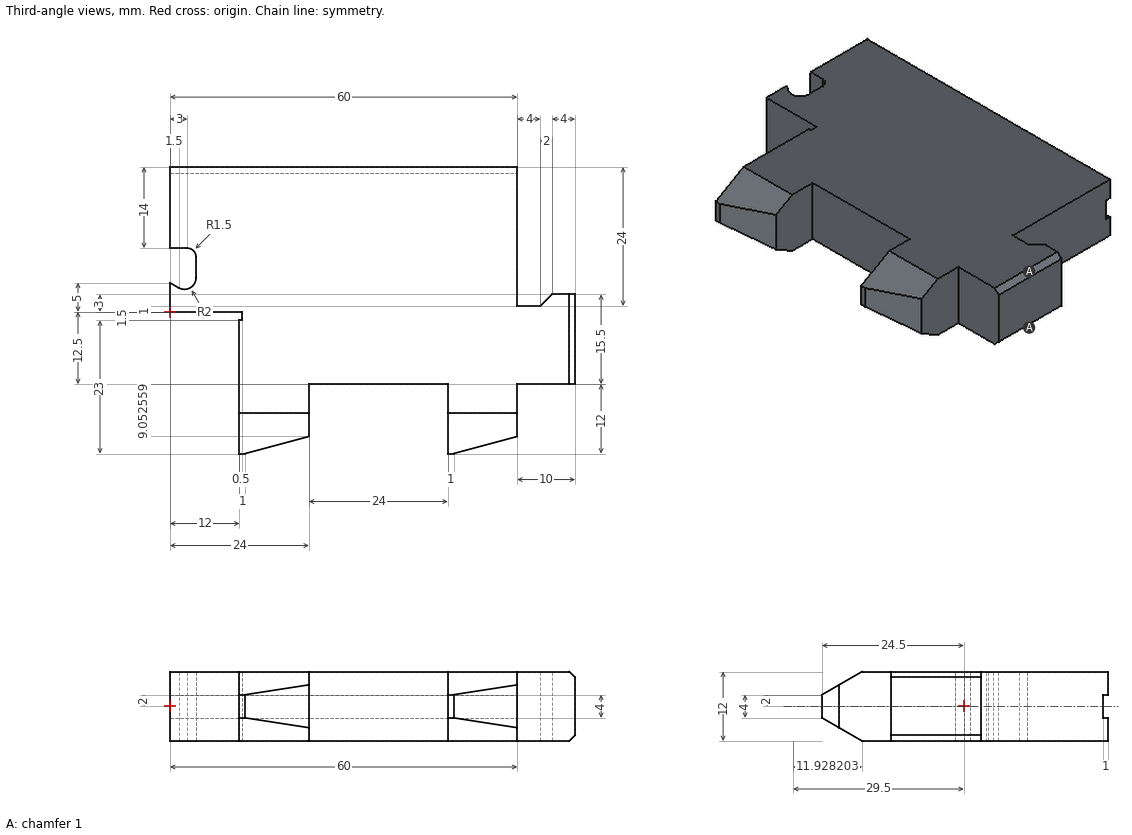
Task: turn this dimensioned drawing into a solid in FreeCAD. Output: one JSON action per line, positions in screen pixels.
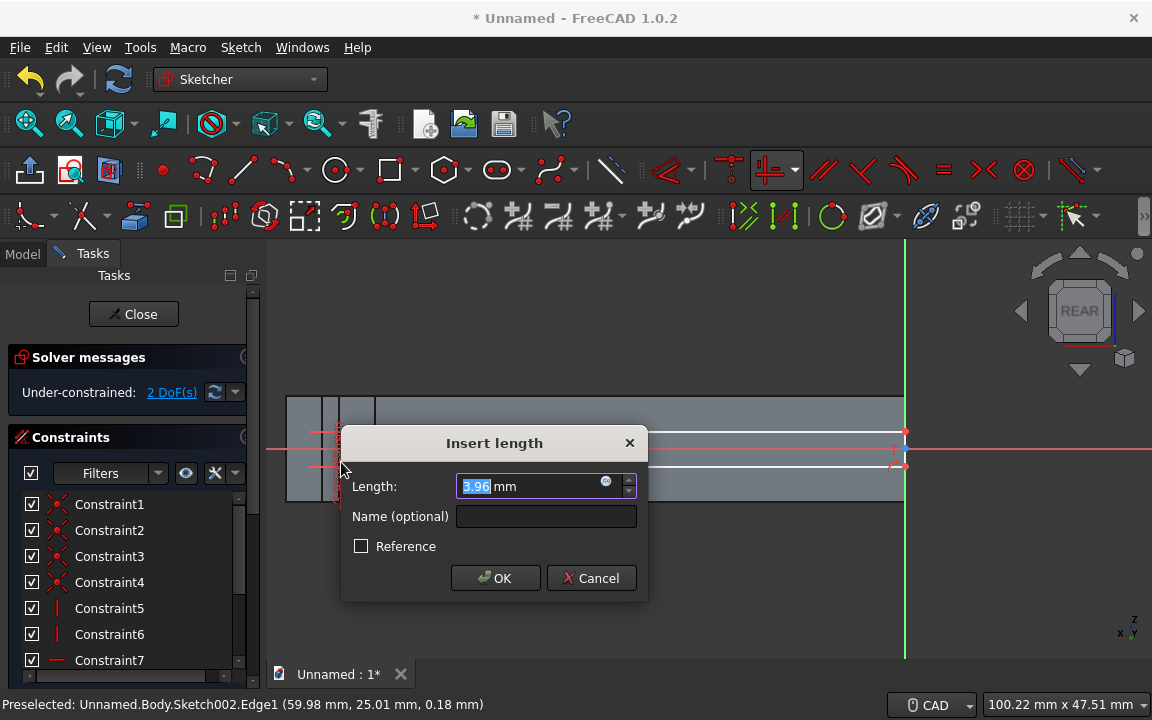
{"action": "type", "text": "4"}
{"action": "key", "text": "Return"}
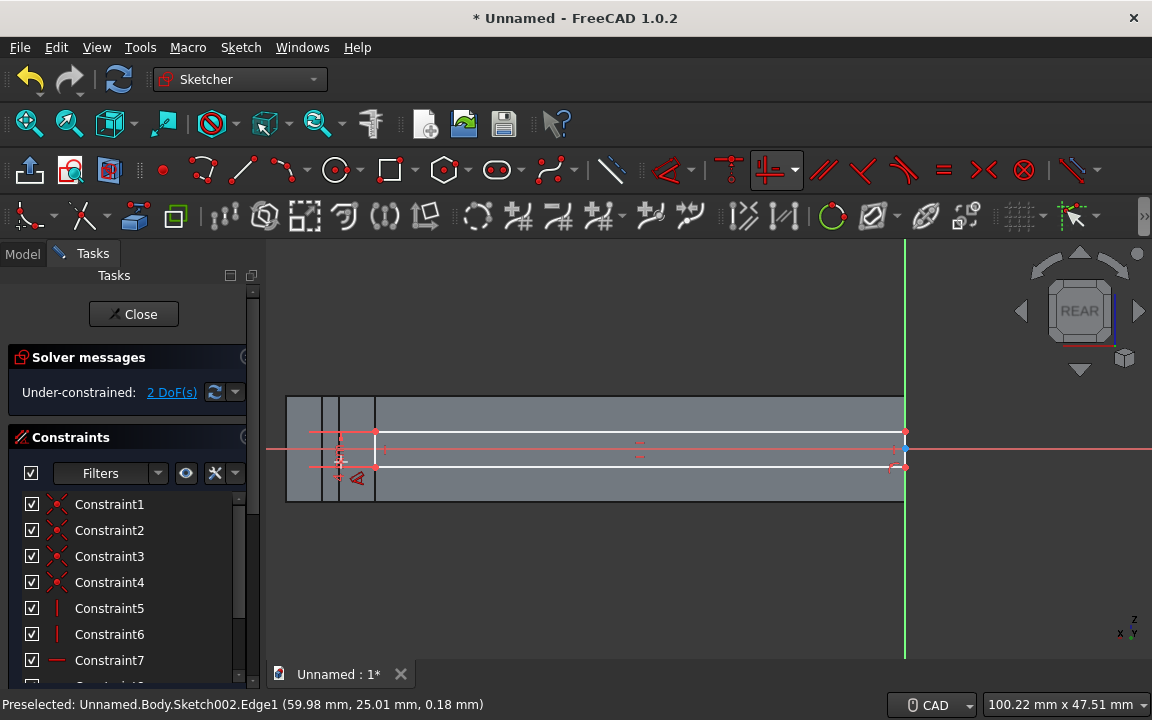
{"action": "left_click", "coordinate": [534, 467]}
{"action": "left_click", "coordinate": [640, 501]}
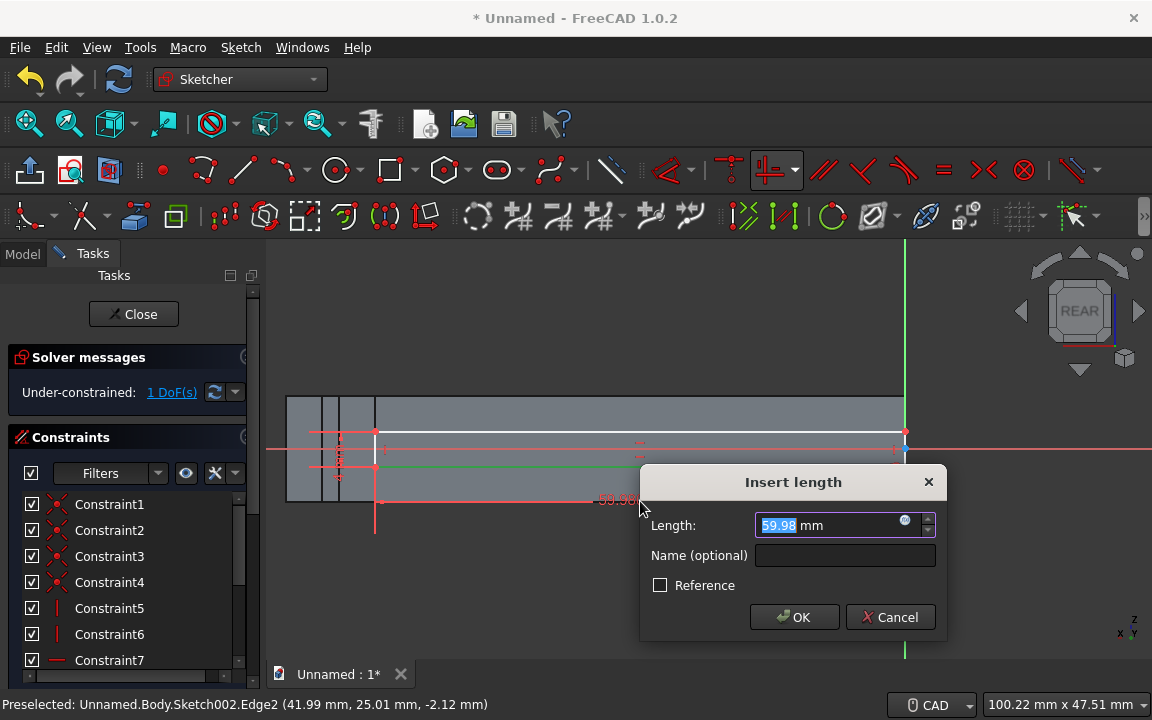
{"action": "type", "text": "60"}
{"action": "key", "text": "Return"}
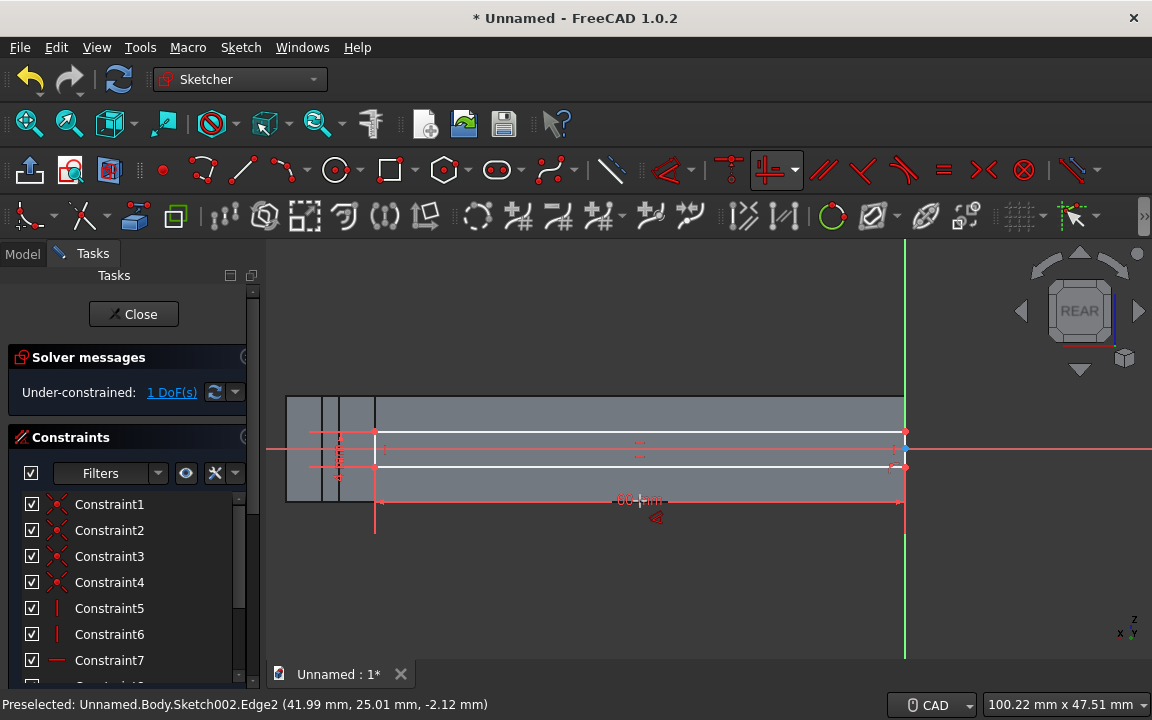
{"action": "scroll", "coordinate": [375, 432], "scroll_direction": "up", "scroll_amount": 5}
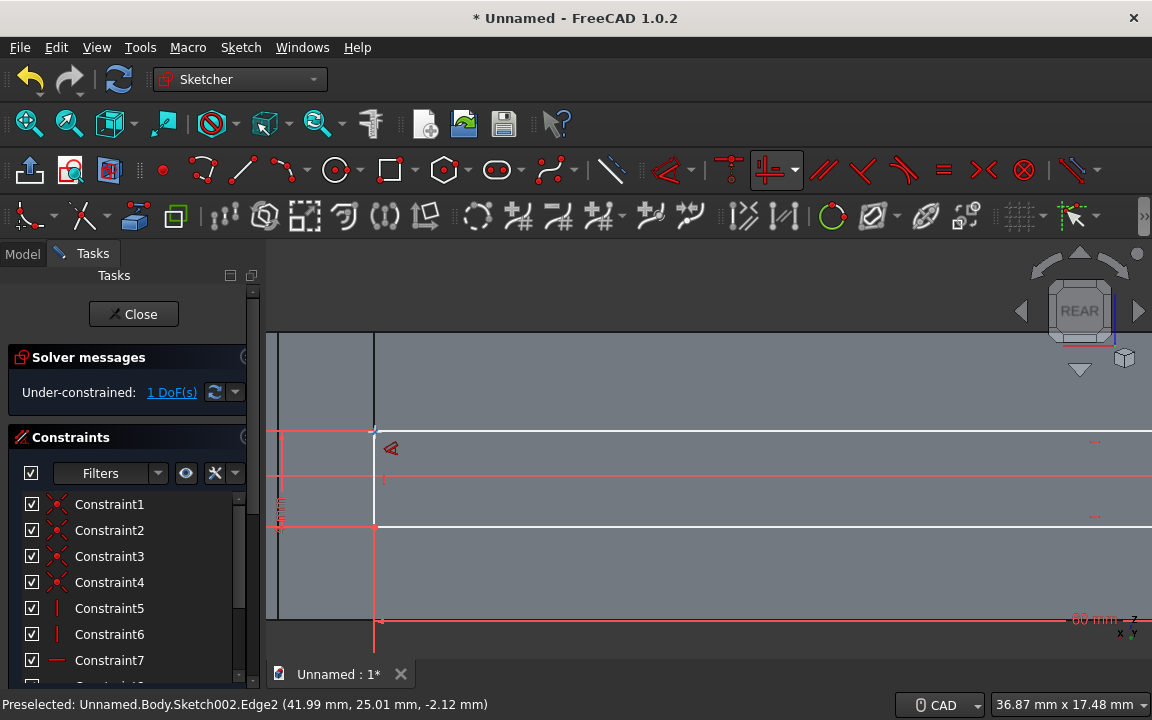
{"action": "left_click", "coordinate": [374, 431]}
{"action": "left_click", "coordinate": [340, 454]}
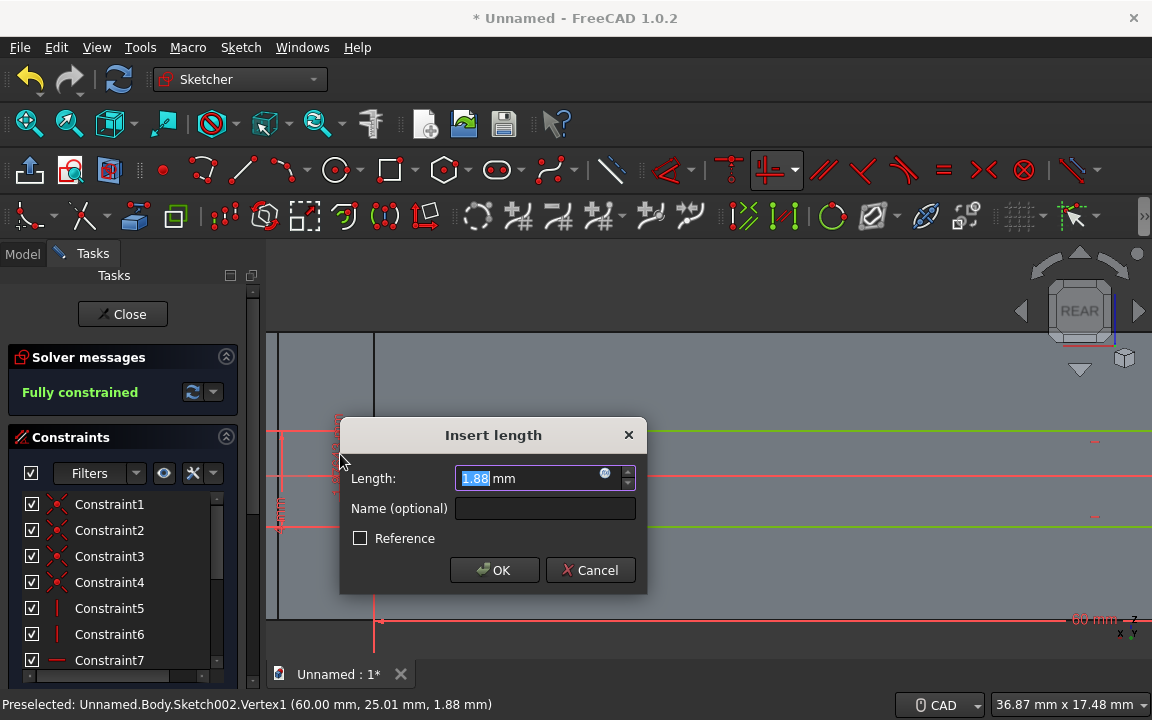
{"action": "type", "text": "2"}
{"action": "key", "text": "Return"}
{"action": "key", "text": "Escape"}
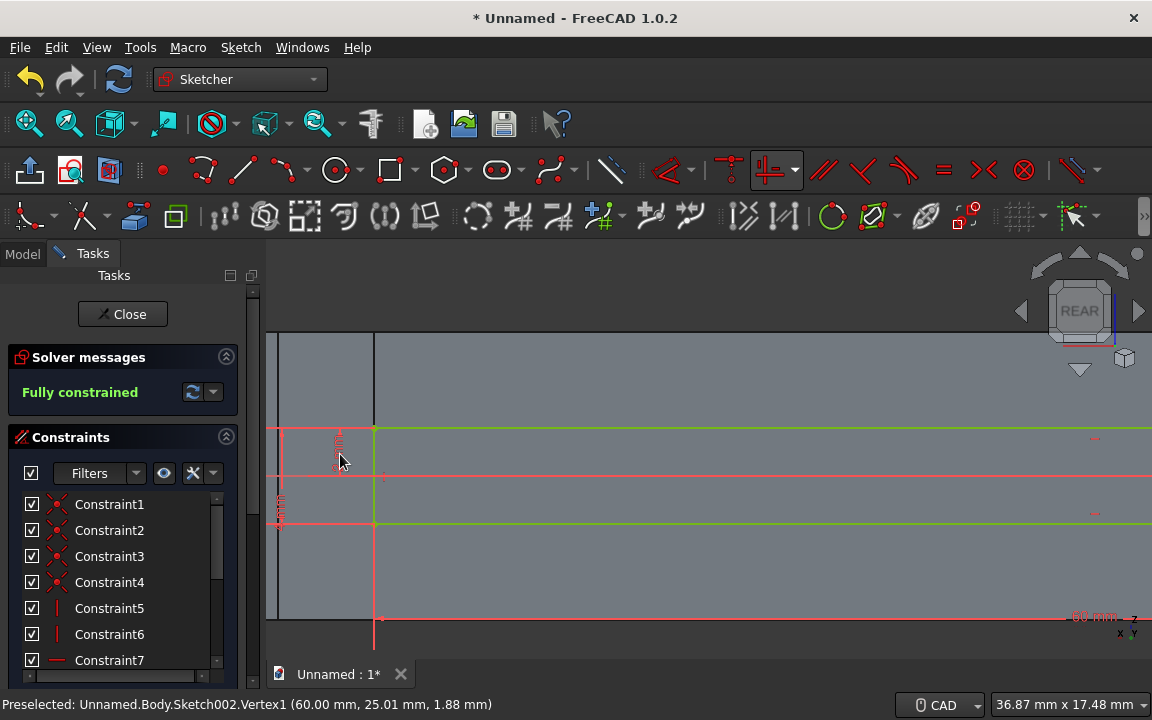
{"action": "left_click", "coordinate": [123, 314]}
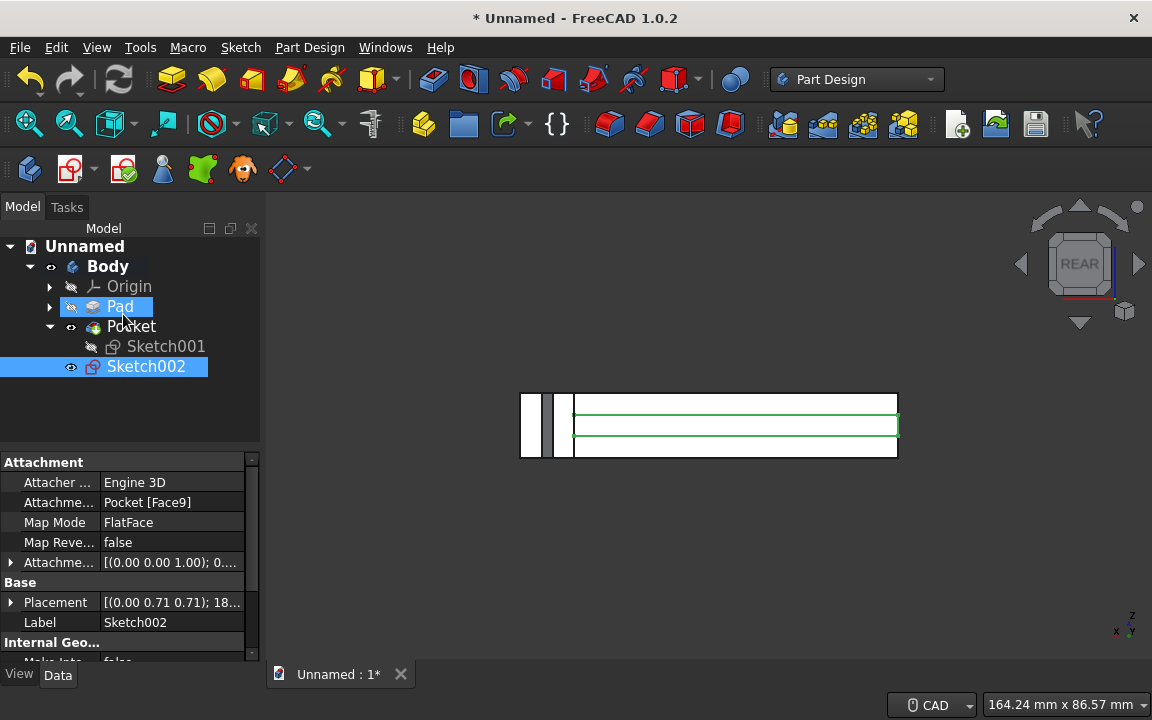
{"action": "left_click", "coordinate": [434, 80]}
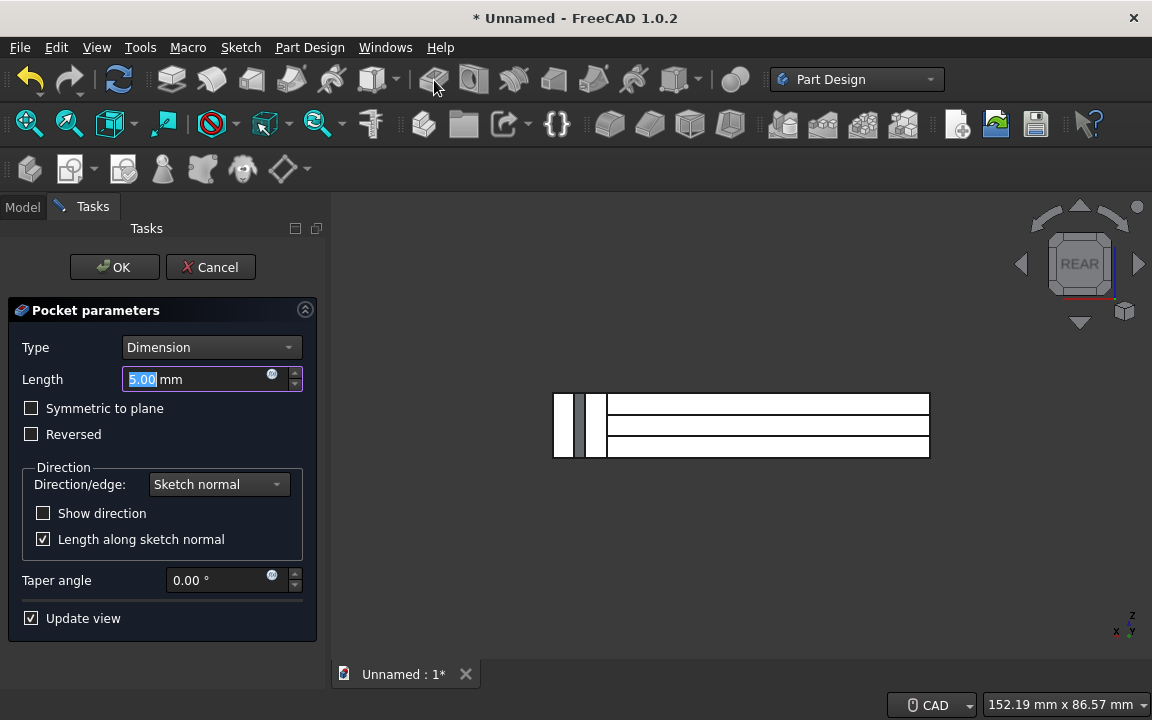
{"action": "type", "text": "1"}
{"action": "key", "text": "Tab"}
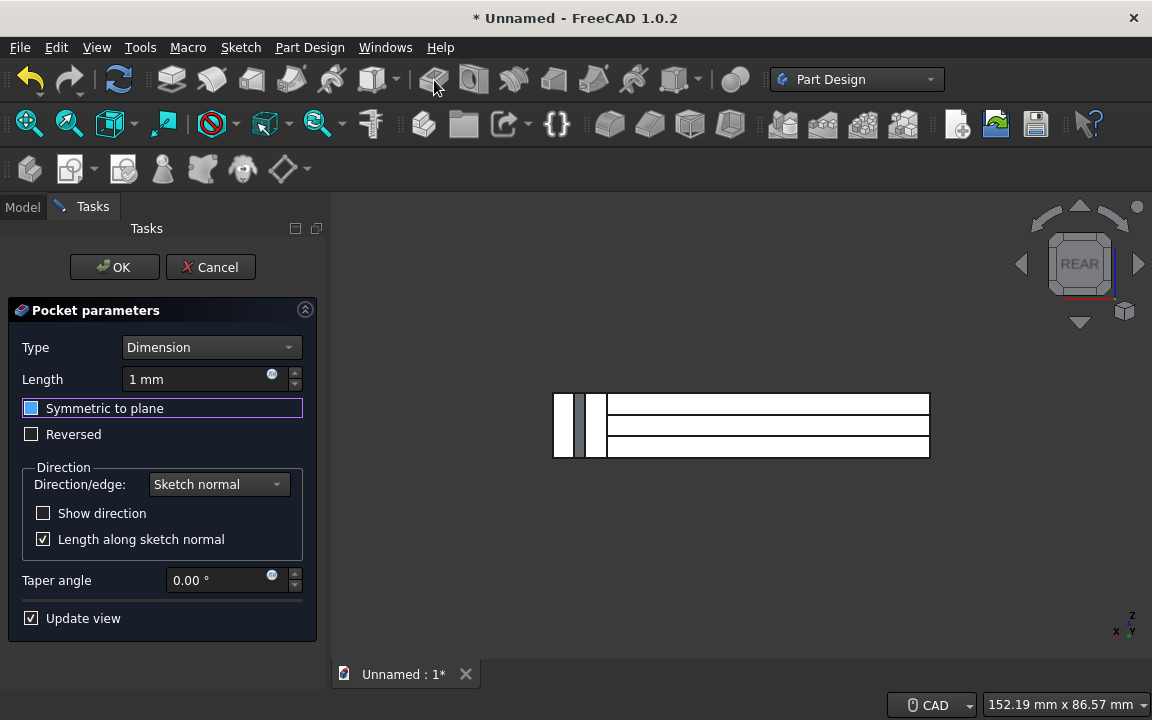
{"action": "left_click", "coordinate": [115, 267]}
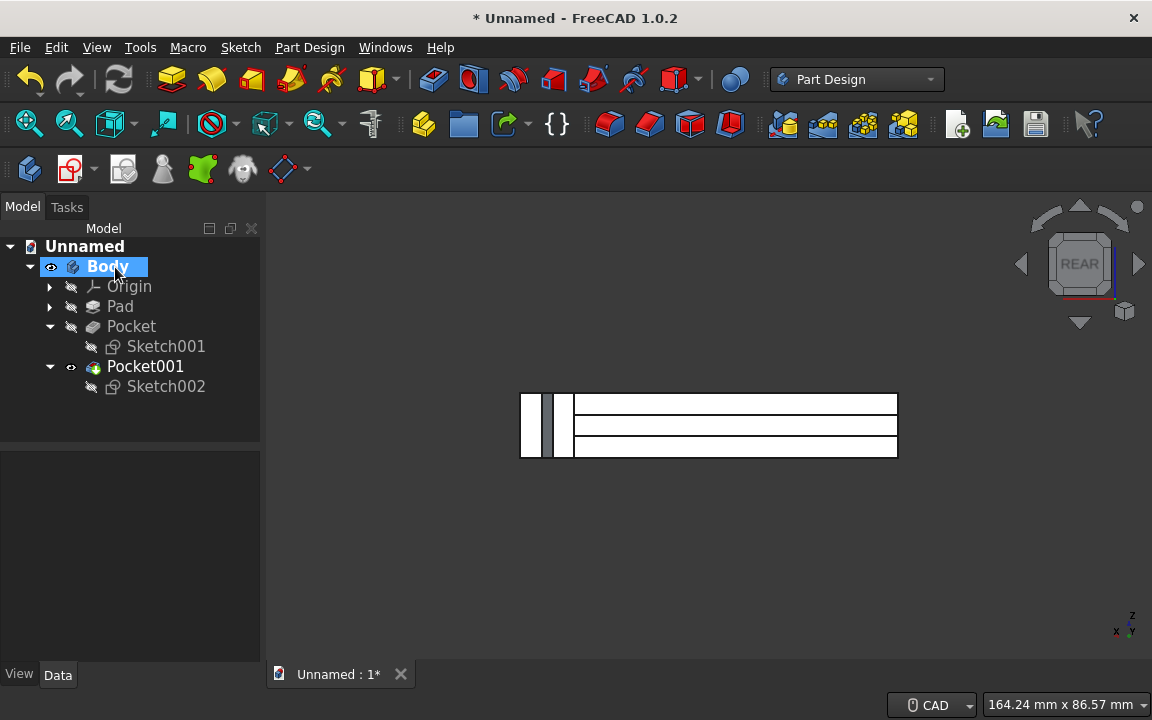
{"action": "left_click", "coordinate": [30, 124]}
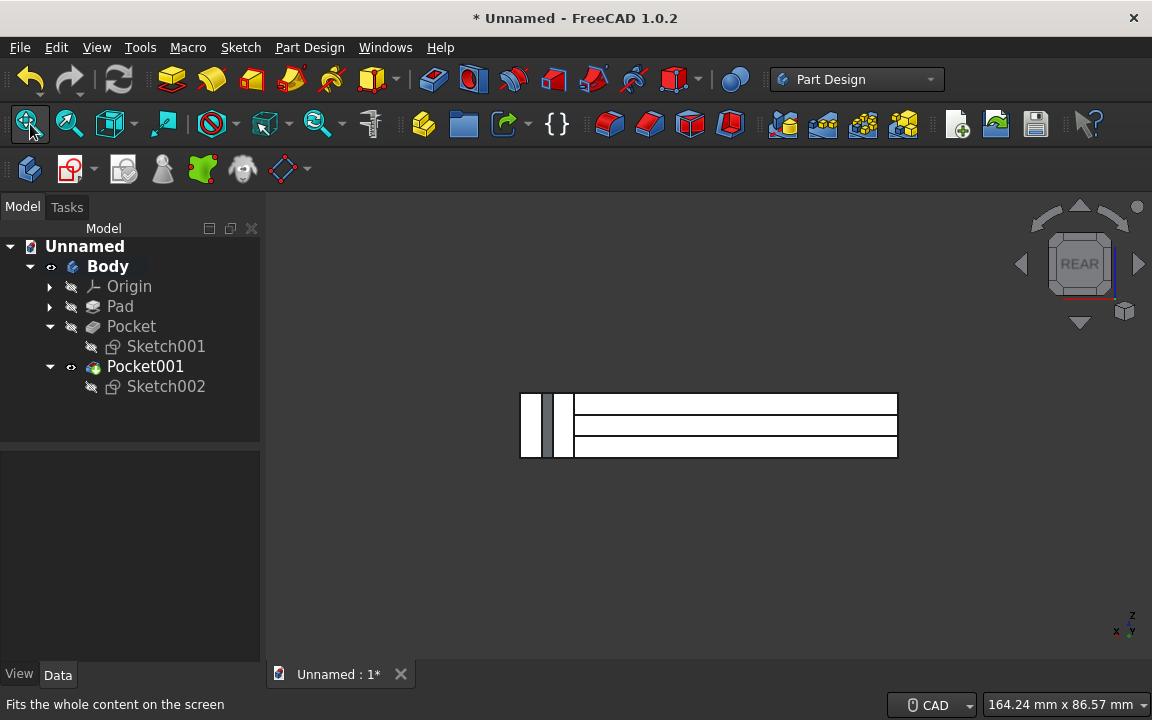
{"action": "key", "text": "0"}